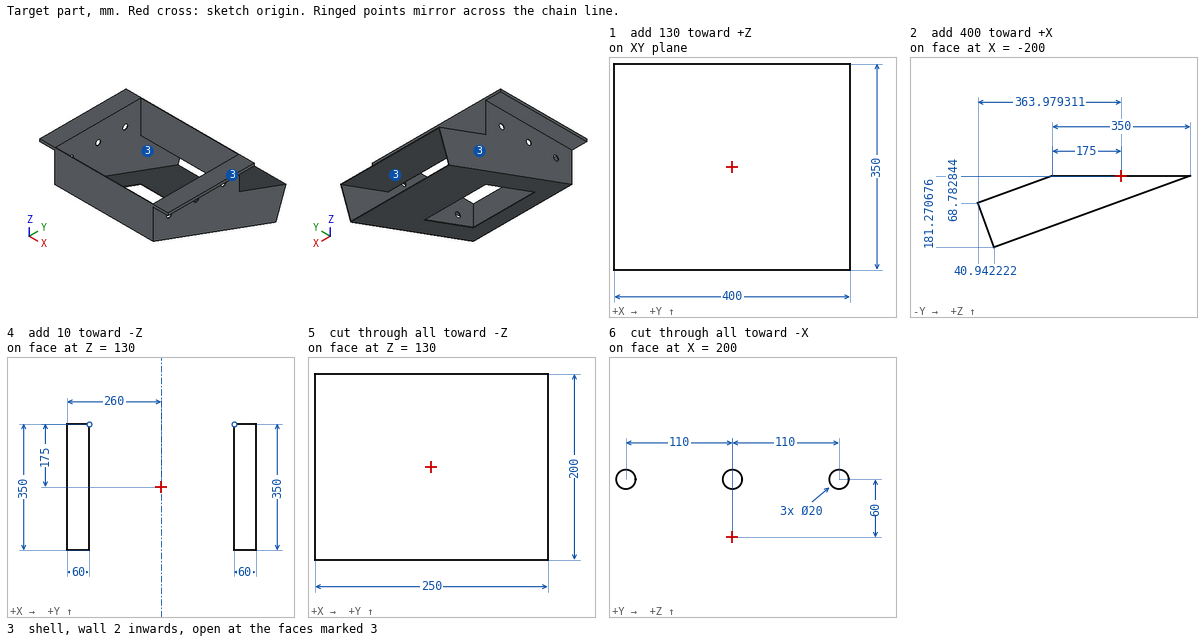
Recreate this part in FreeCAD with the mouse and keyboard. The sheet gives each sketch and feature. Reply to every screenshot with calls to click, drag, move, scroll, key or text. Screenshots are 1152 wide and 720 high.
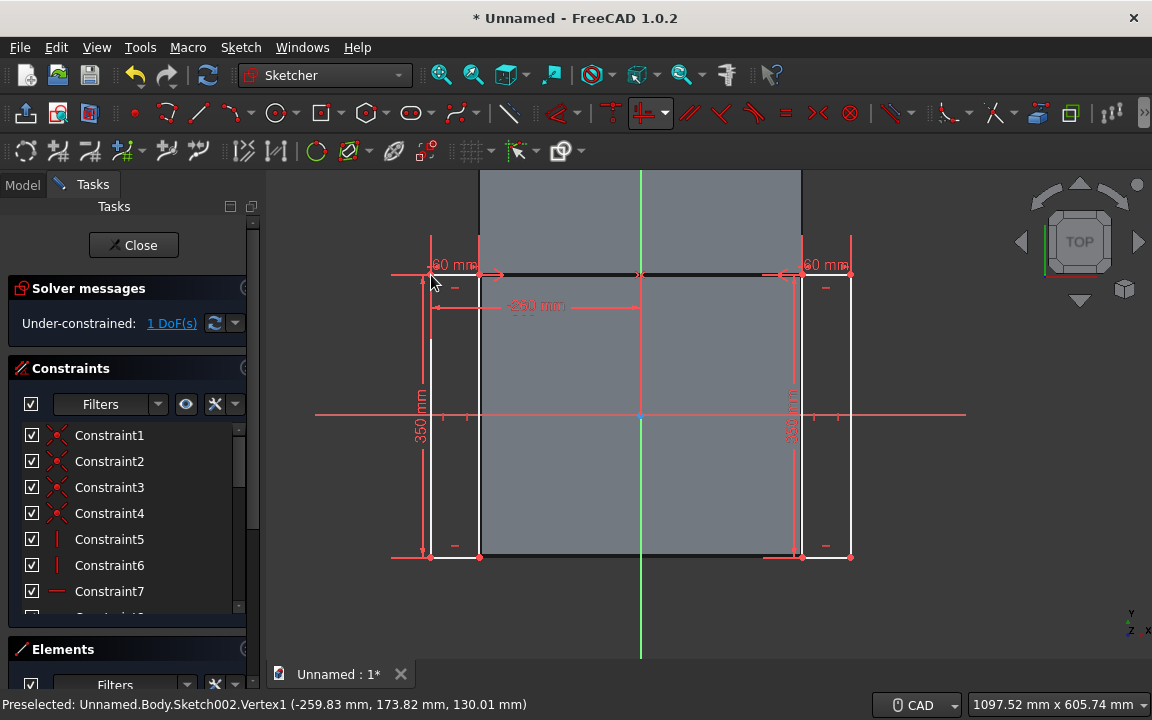
click(431, 275)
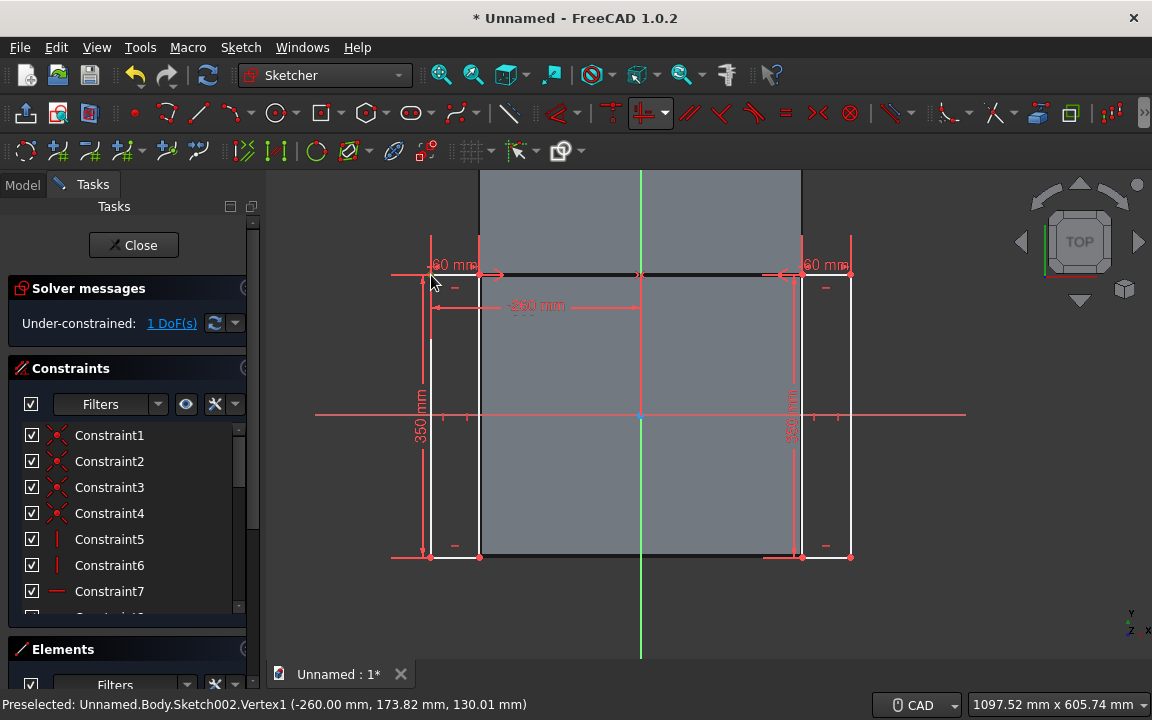
click(580, 114)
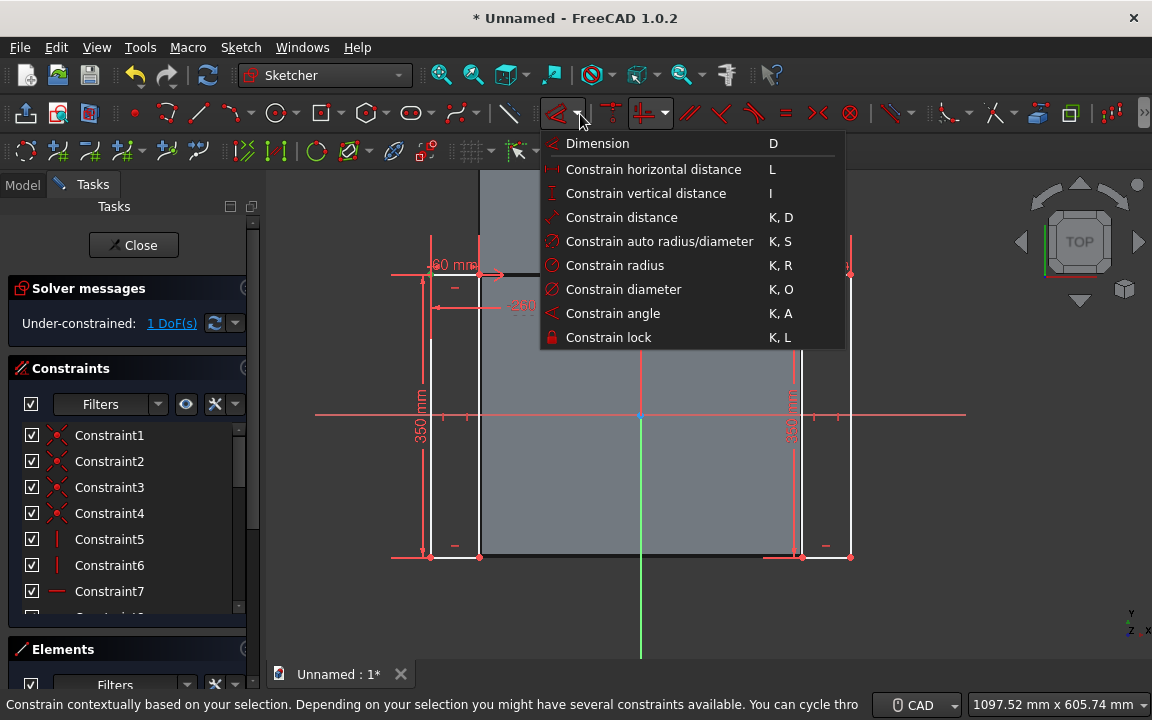
click(693, 193)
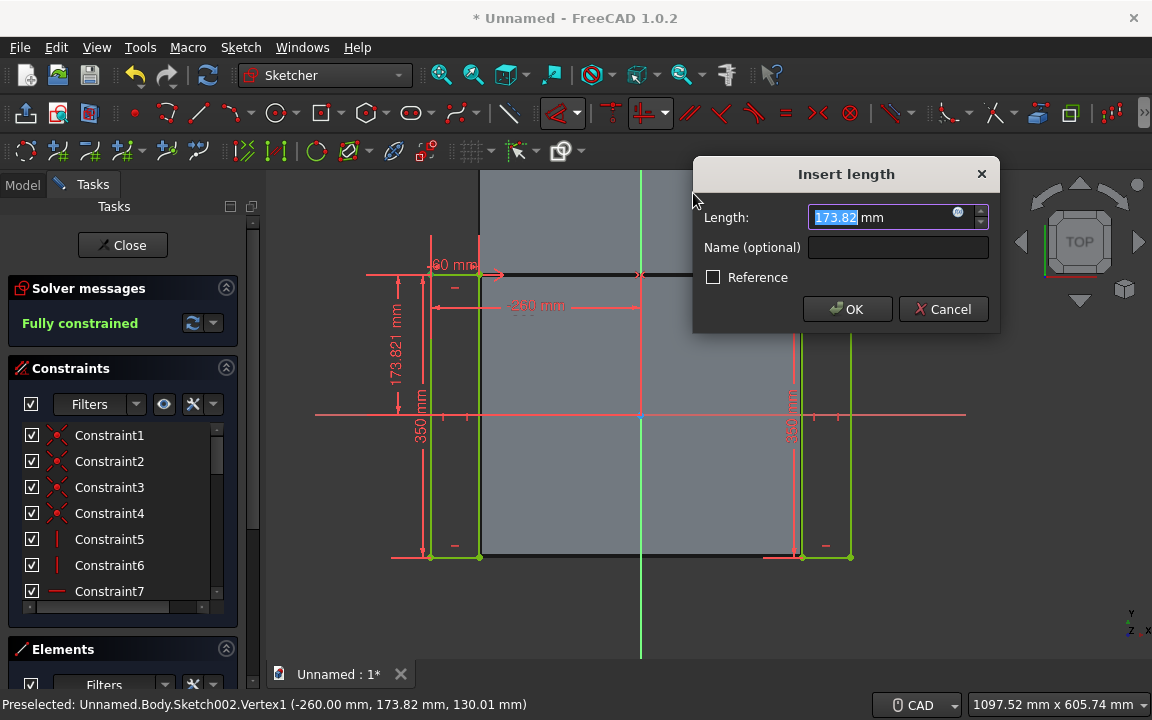
text(175)
key(Return)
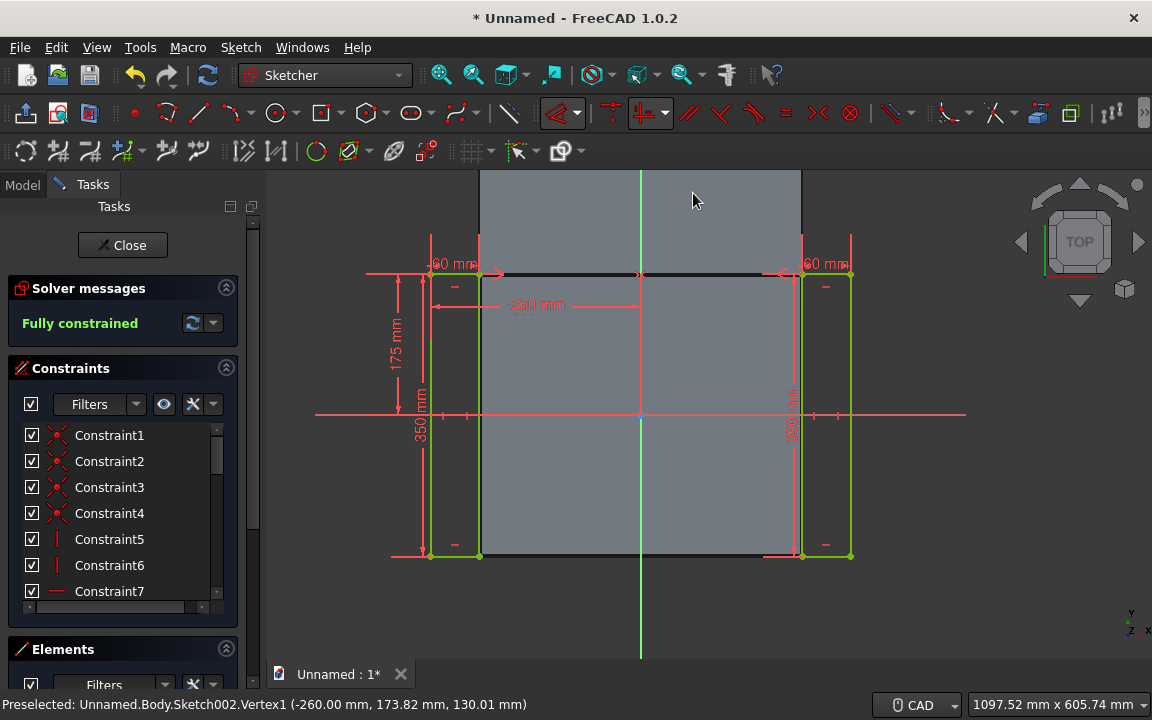
click(123, 245)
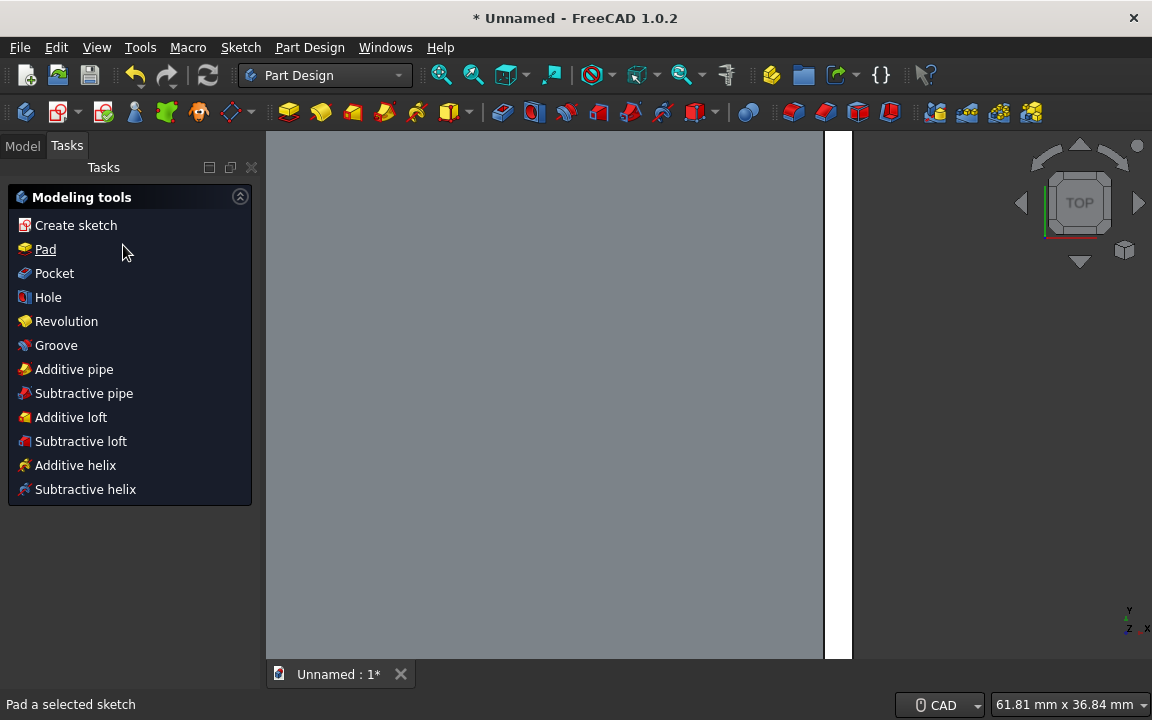
click(290, 112)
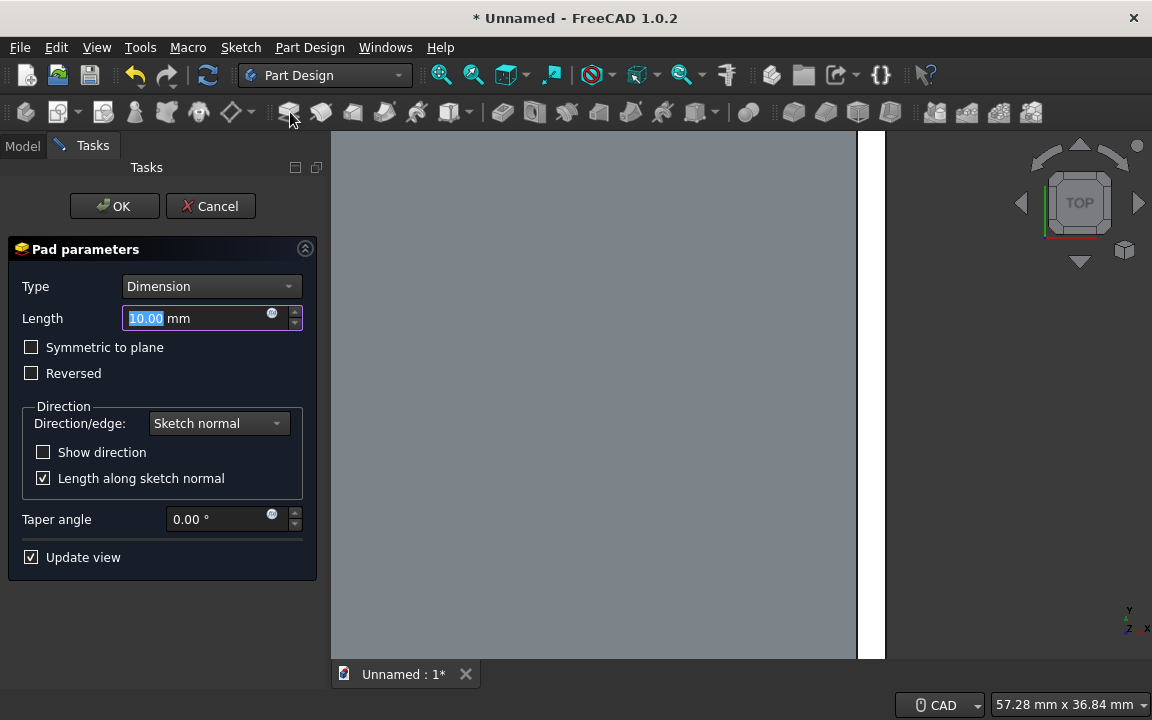
text(10)
key(Tab)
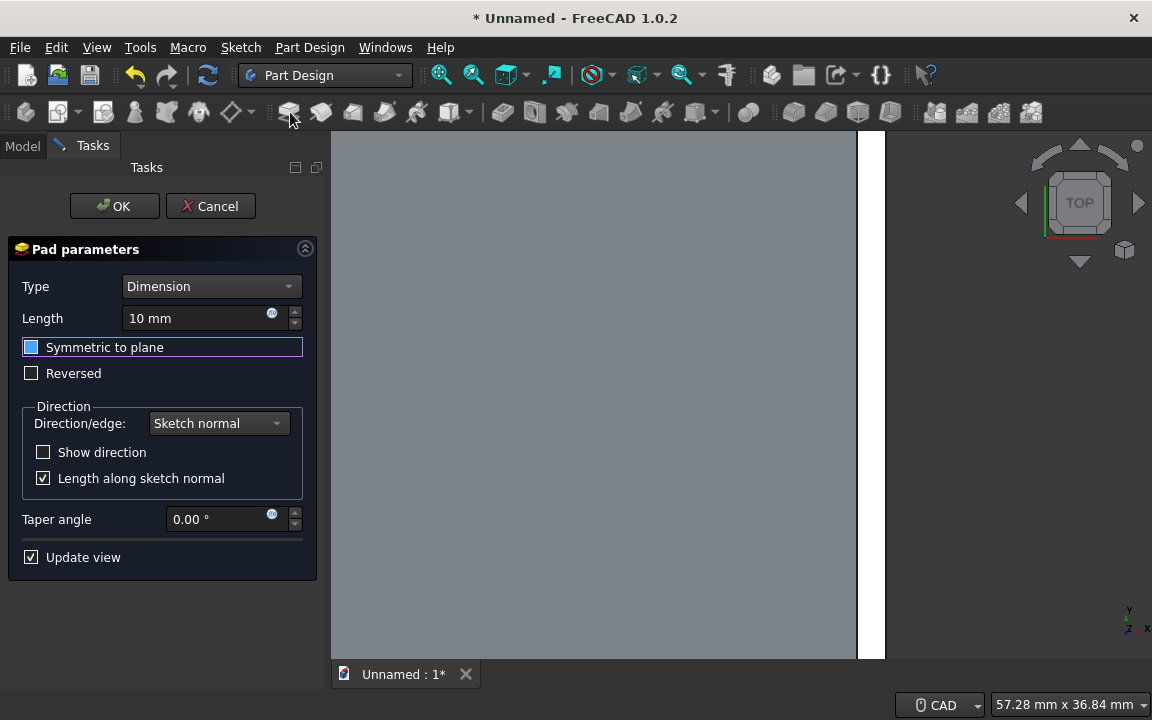
click(30, 373)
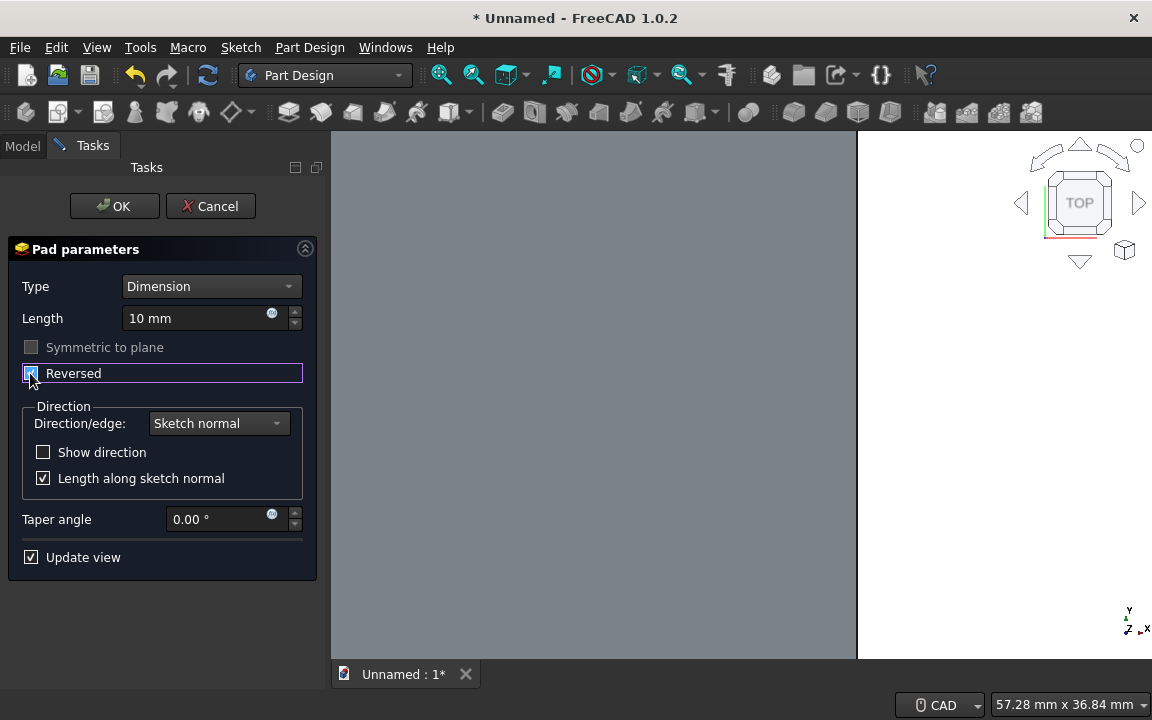
click(115, 206)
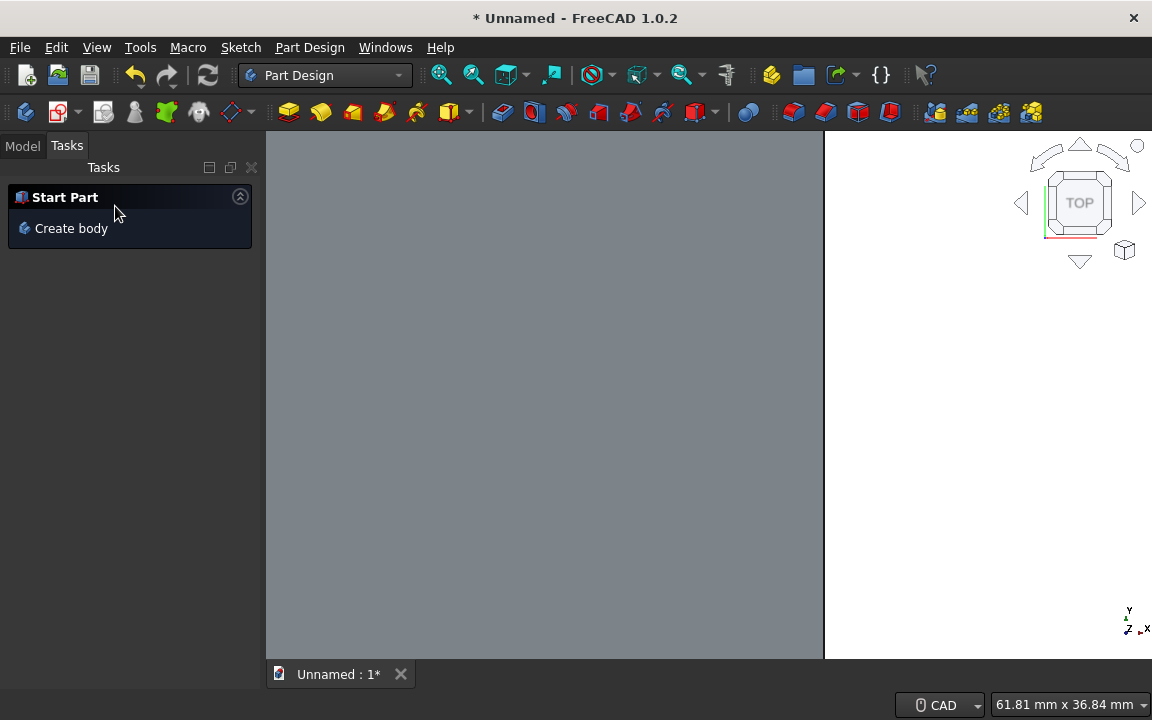
click(442, 76)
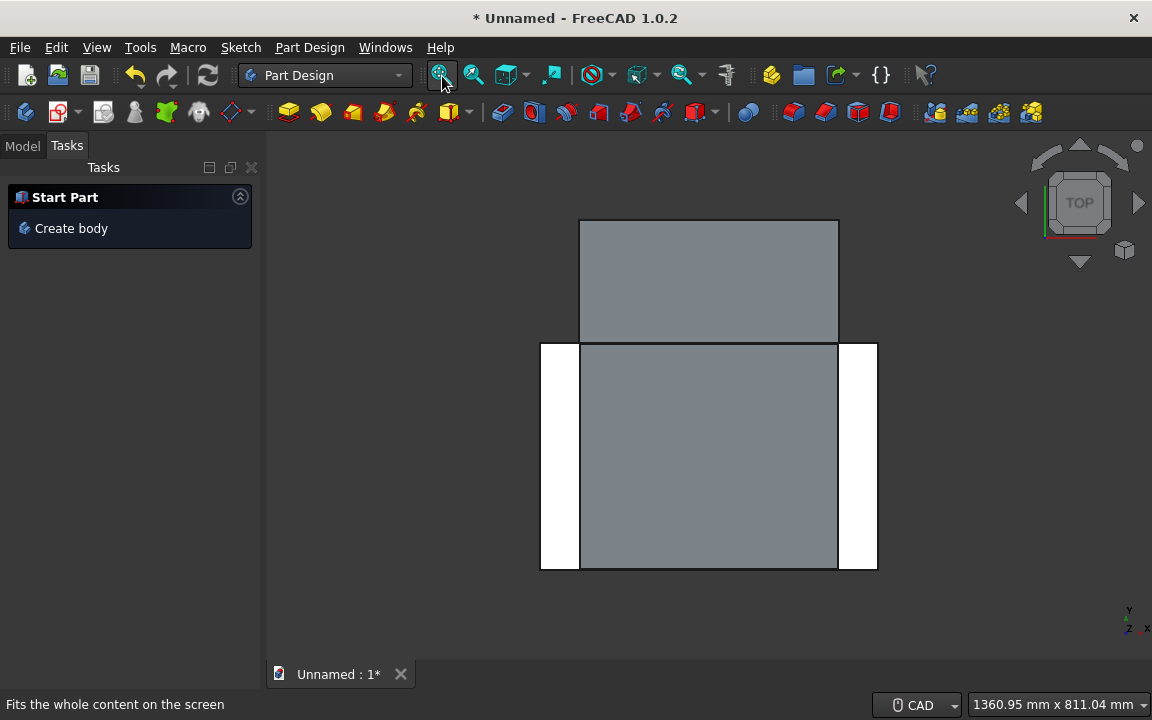
click(564, 358)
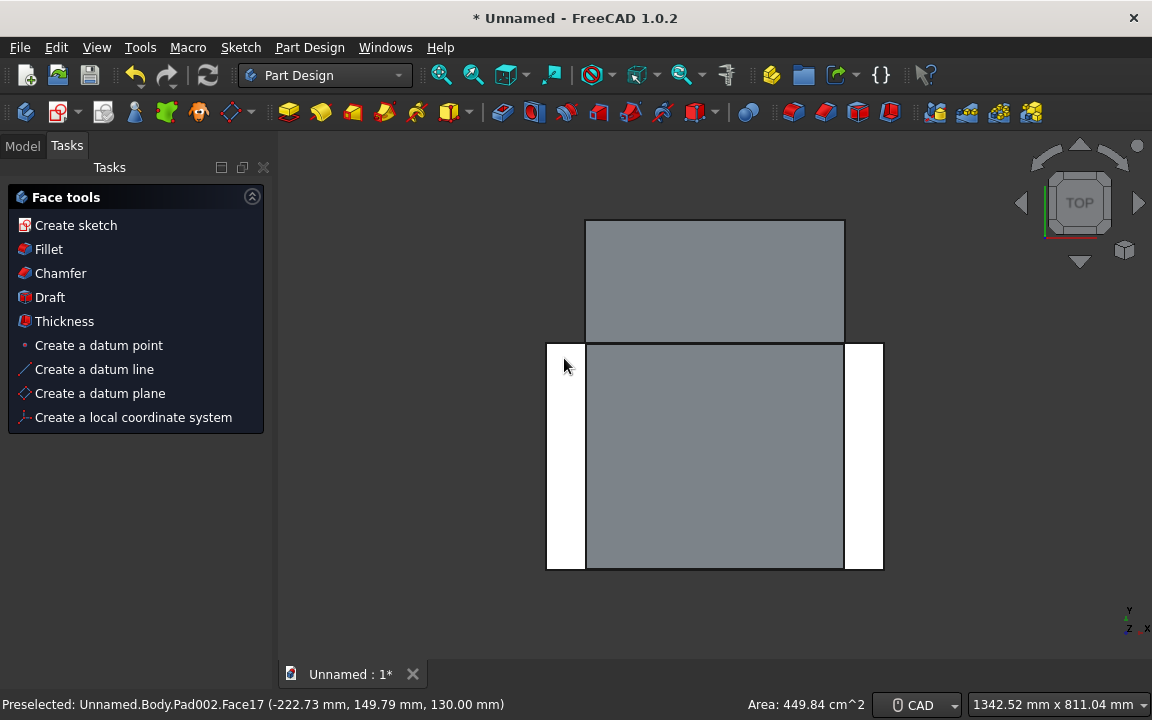
click(58, 112)